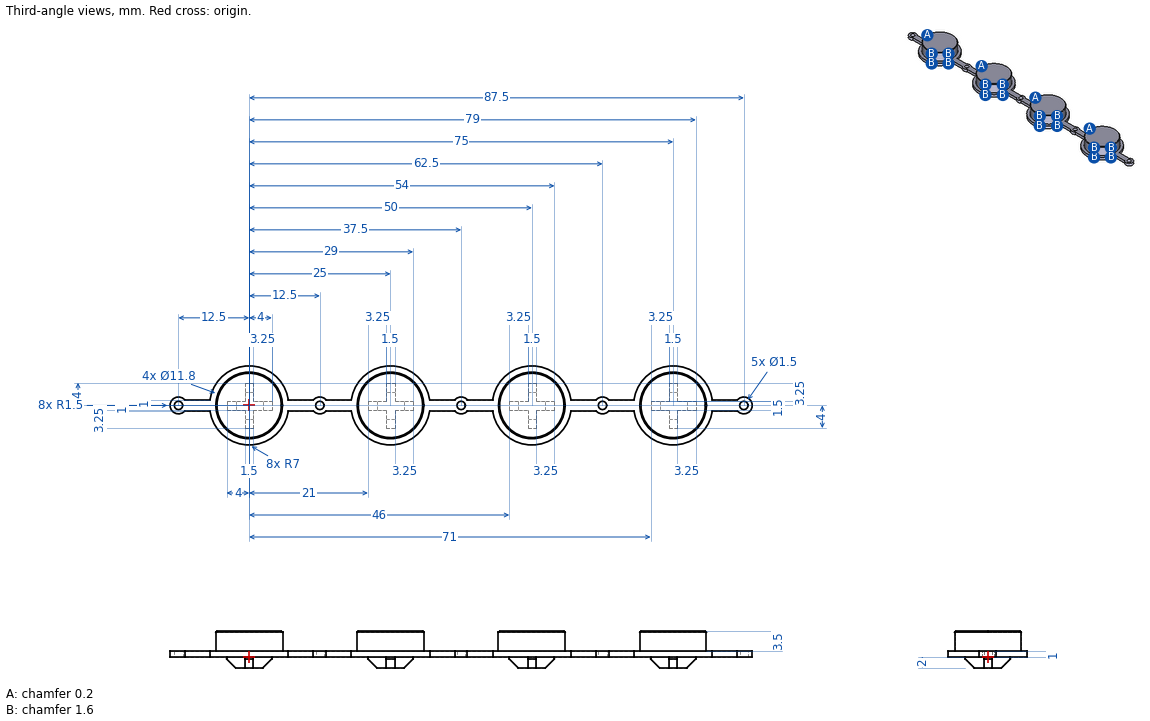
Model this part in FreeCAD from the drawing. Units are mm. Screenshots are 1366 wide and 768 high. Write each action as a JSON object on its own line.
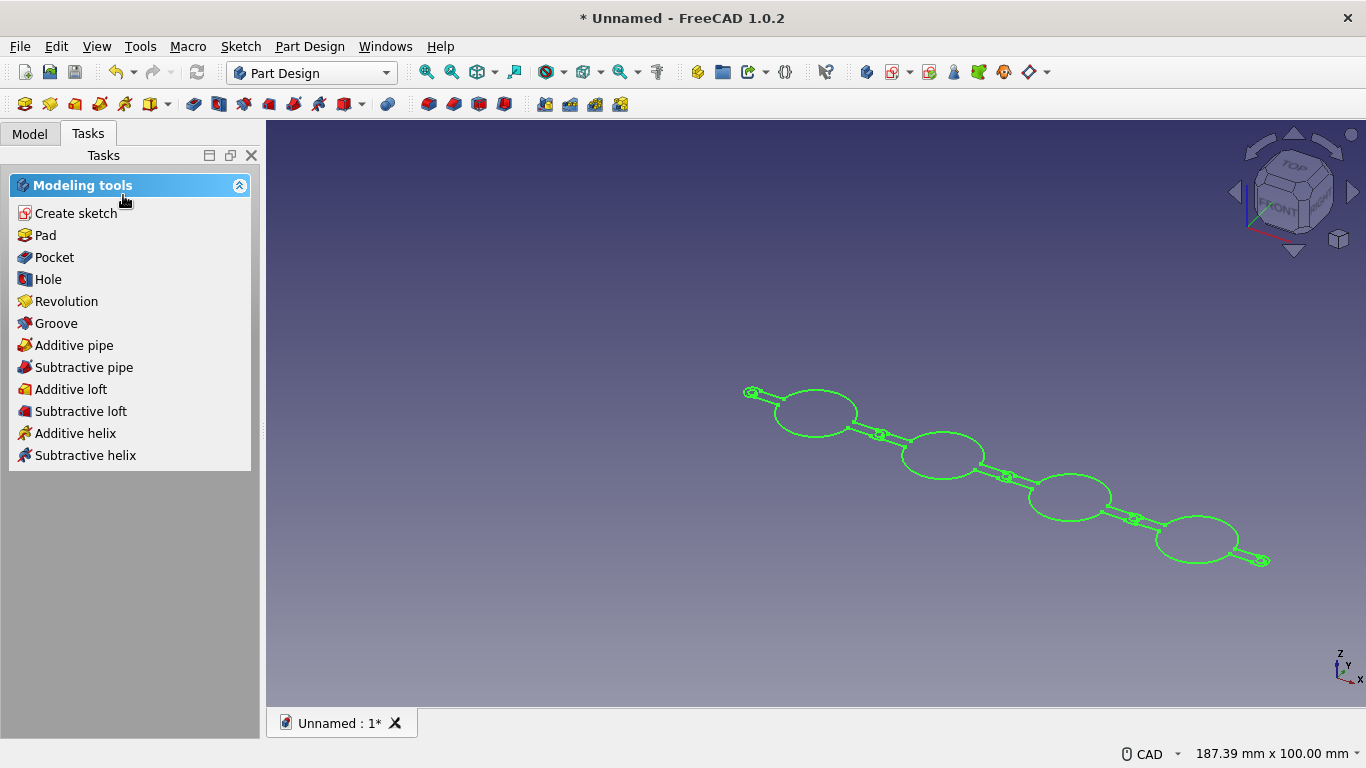
{"action": "left_click", "coordinate": [25, 104]}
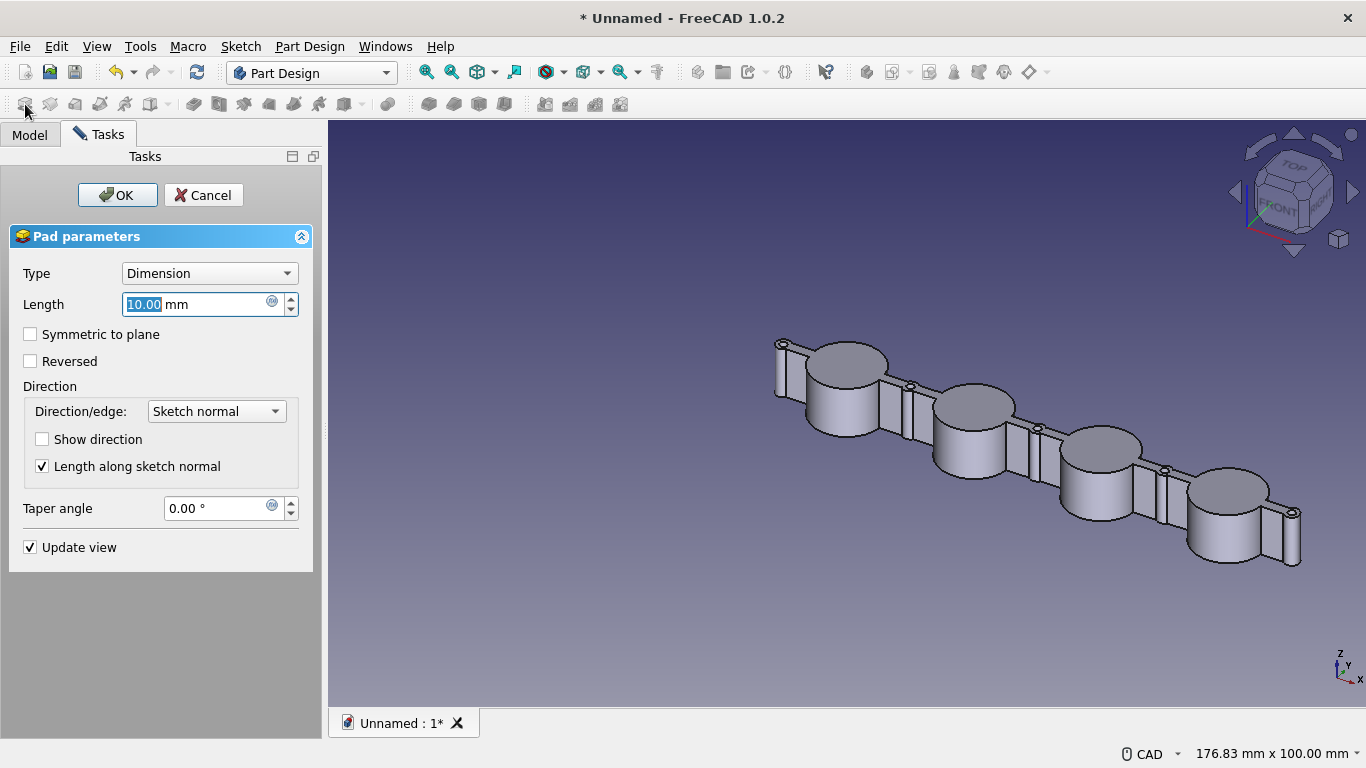
{"action": "type", "text": "1"}
{"action": "key", "text": "Tab"}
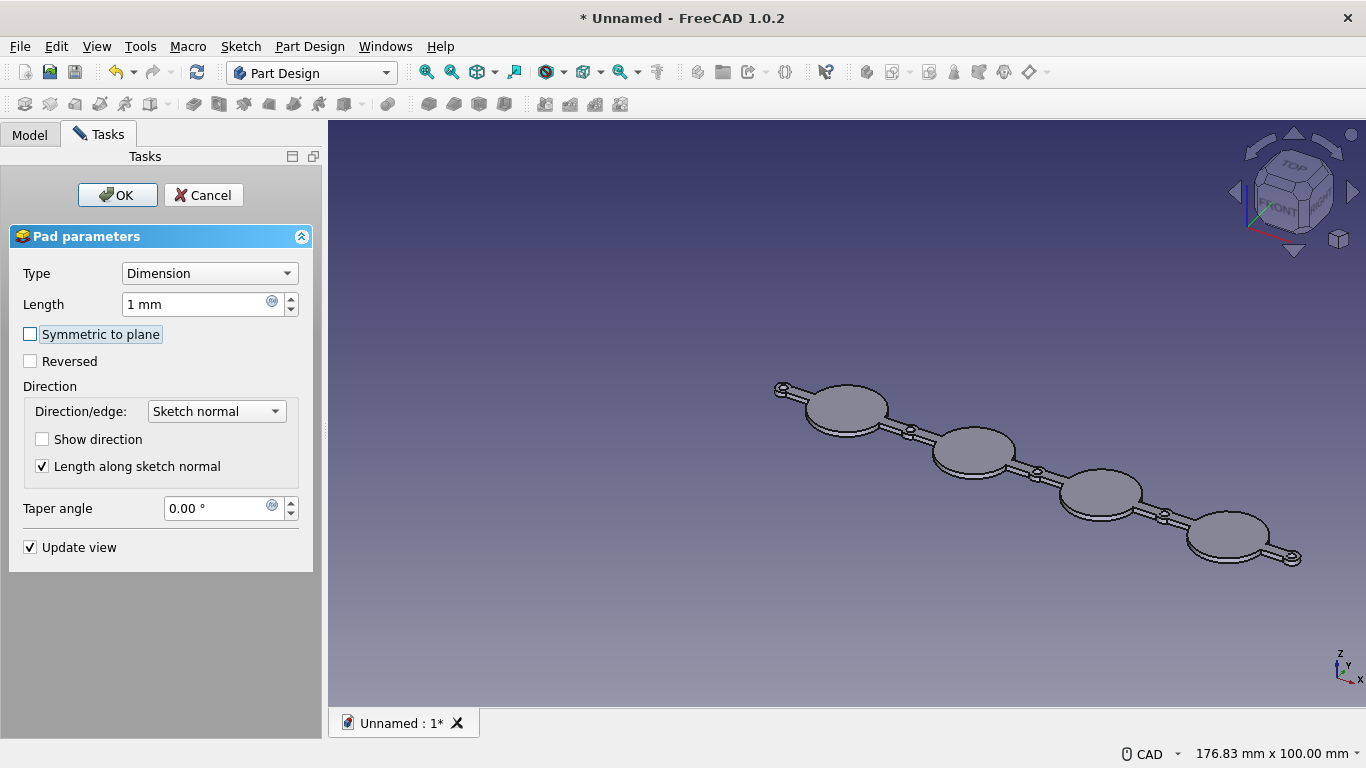
{"action": "left_click", "coordinate": [118, 195]}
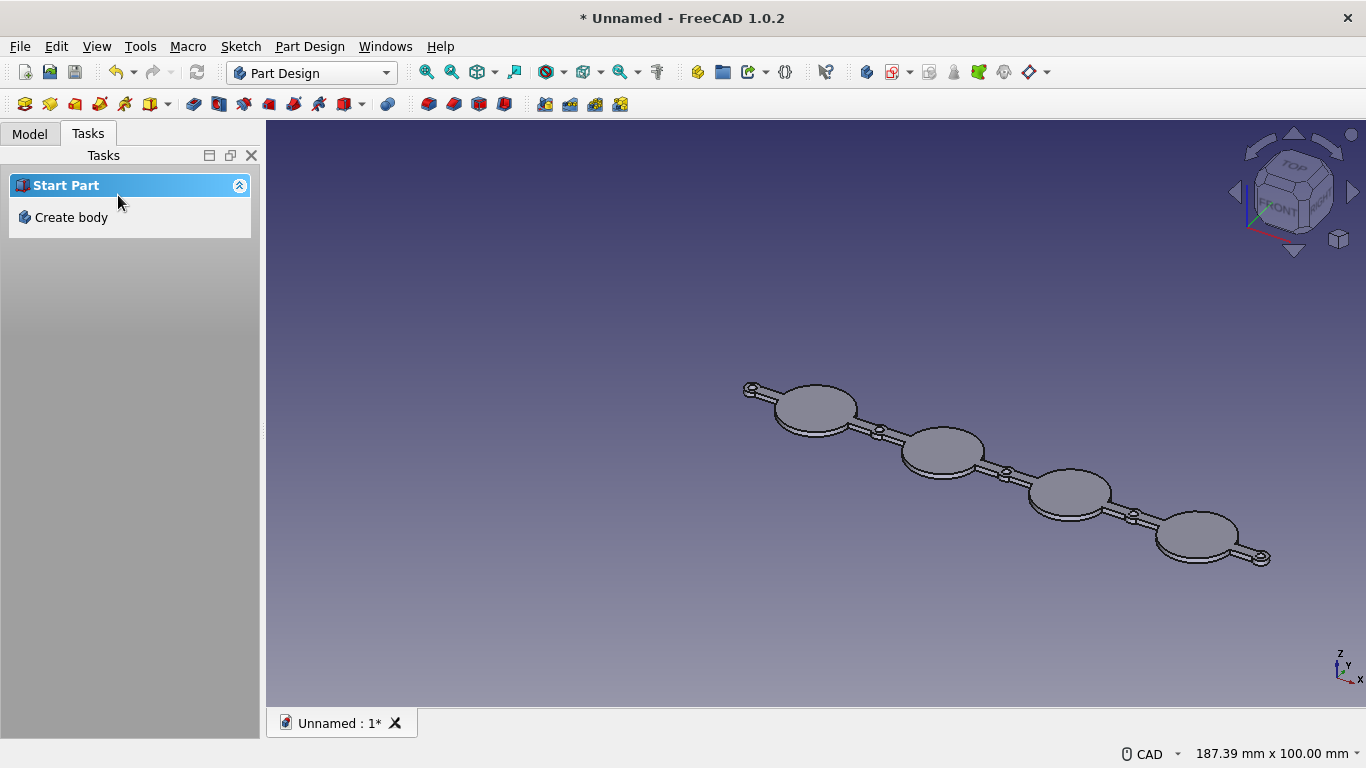
{"action": "left_click", "coordinate": [1081, 496]}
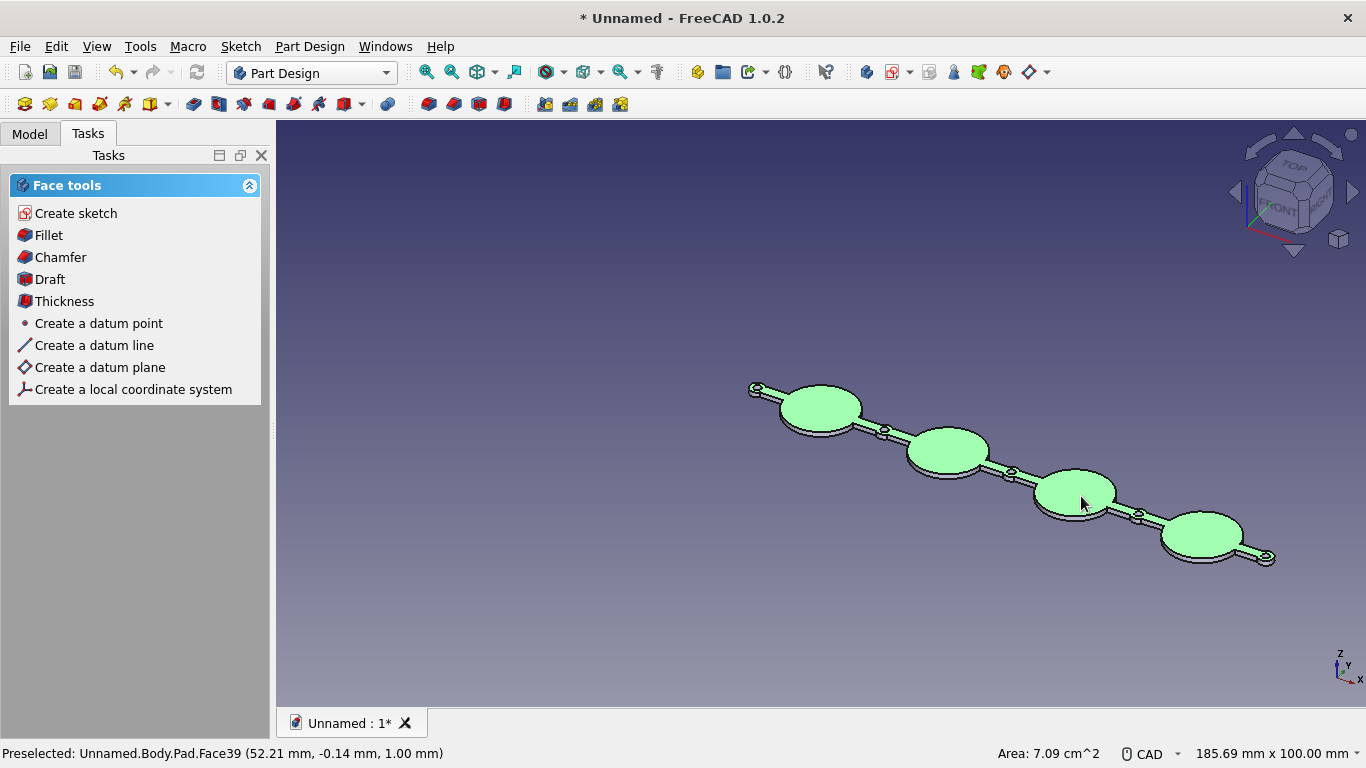
{"action": "left_click", "coordinate": [892, 72]}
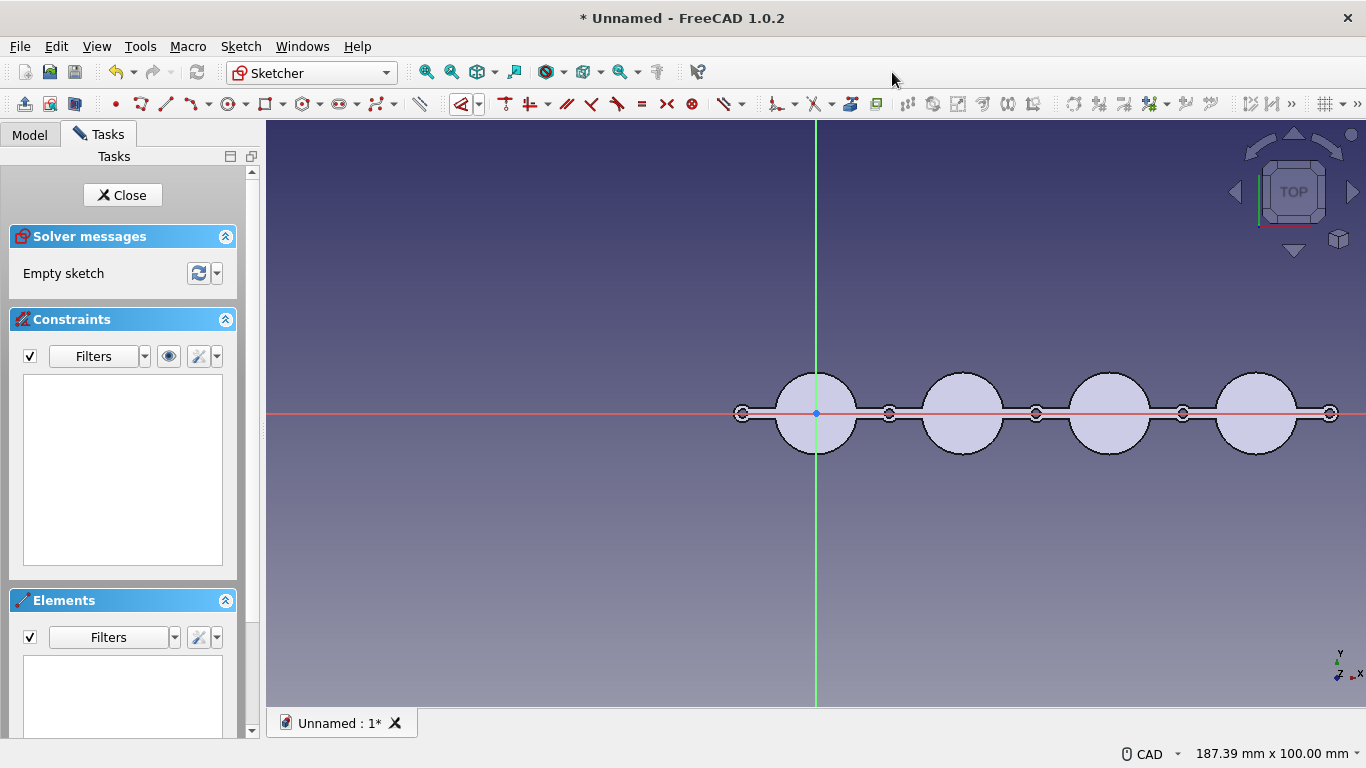
{"action": "scroll", "coordinate": [294, 413], "scroll_direction": "down", "scroll_amount": 1}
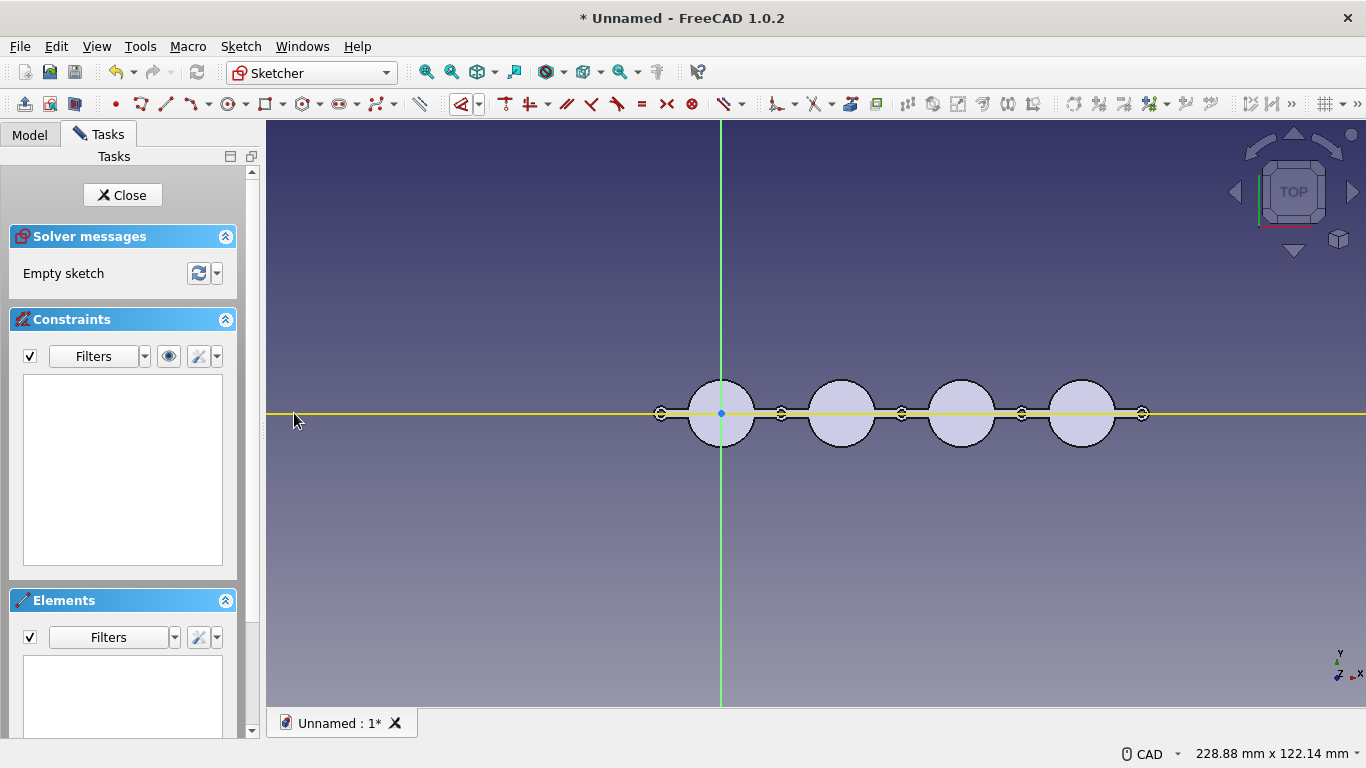
{"action": "scroll", "coordinate": [1201, 413], "scroll_direction": "up", "scroll_amount": 2}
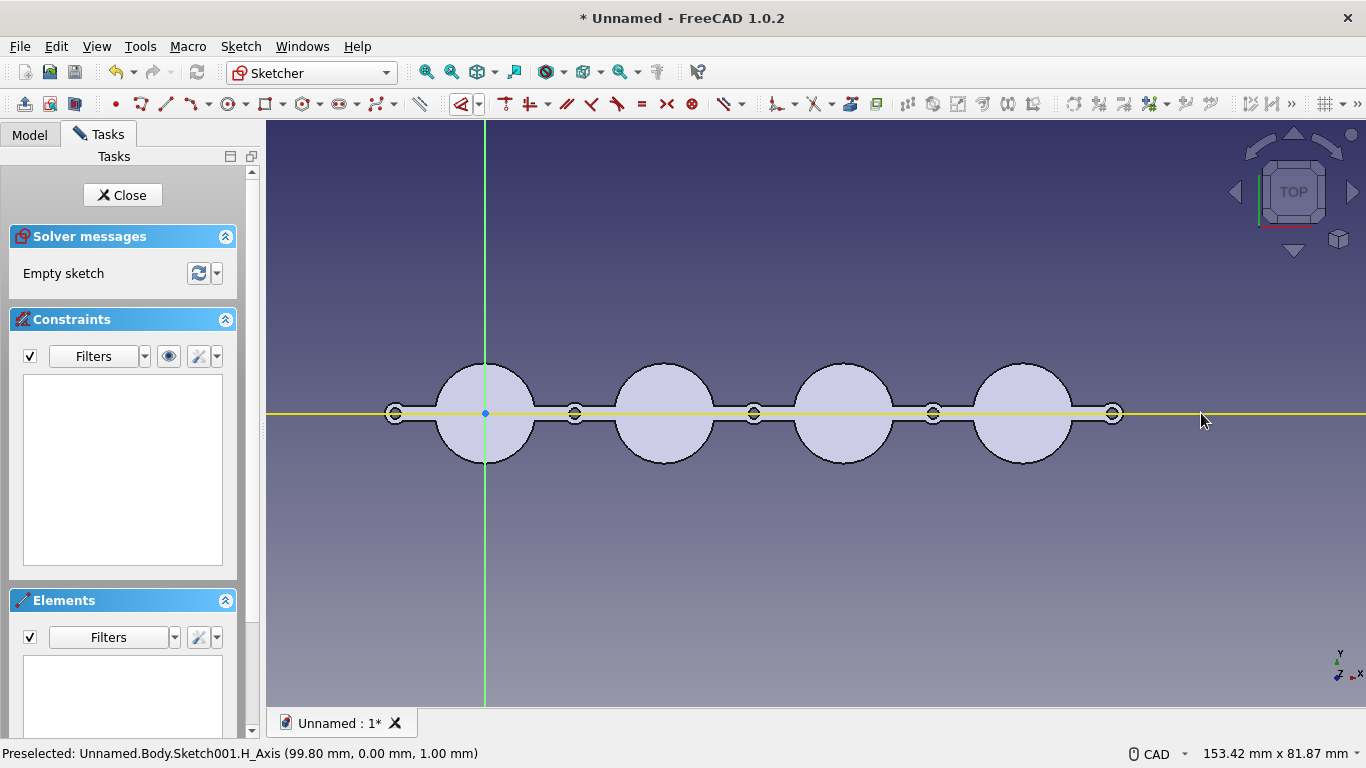
{"action": "key", "text": "g c"}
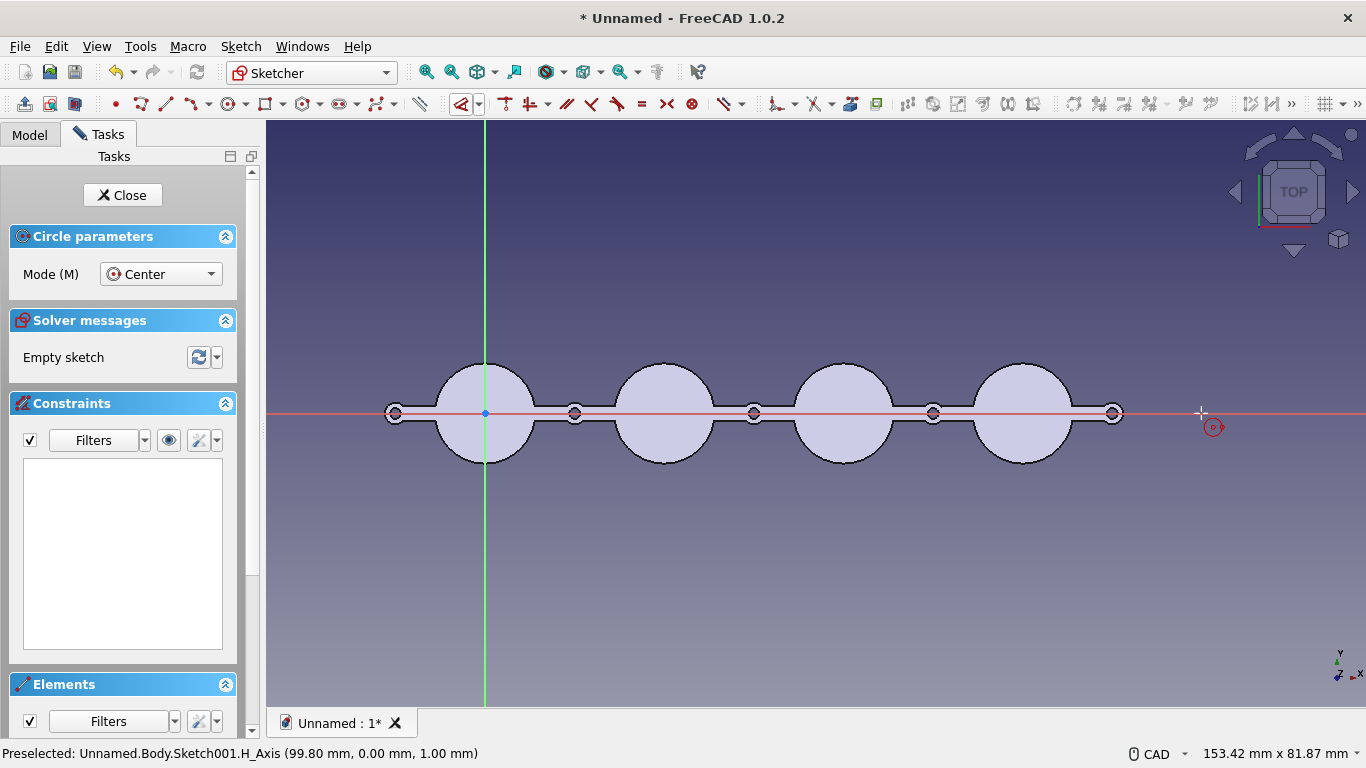
{"action": "left_click", "coordinate": [485, 414]}
{"action": "left_click", "coordinate": [515, 384]}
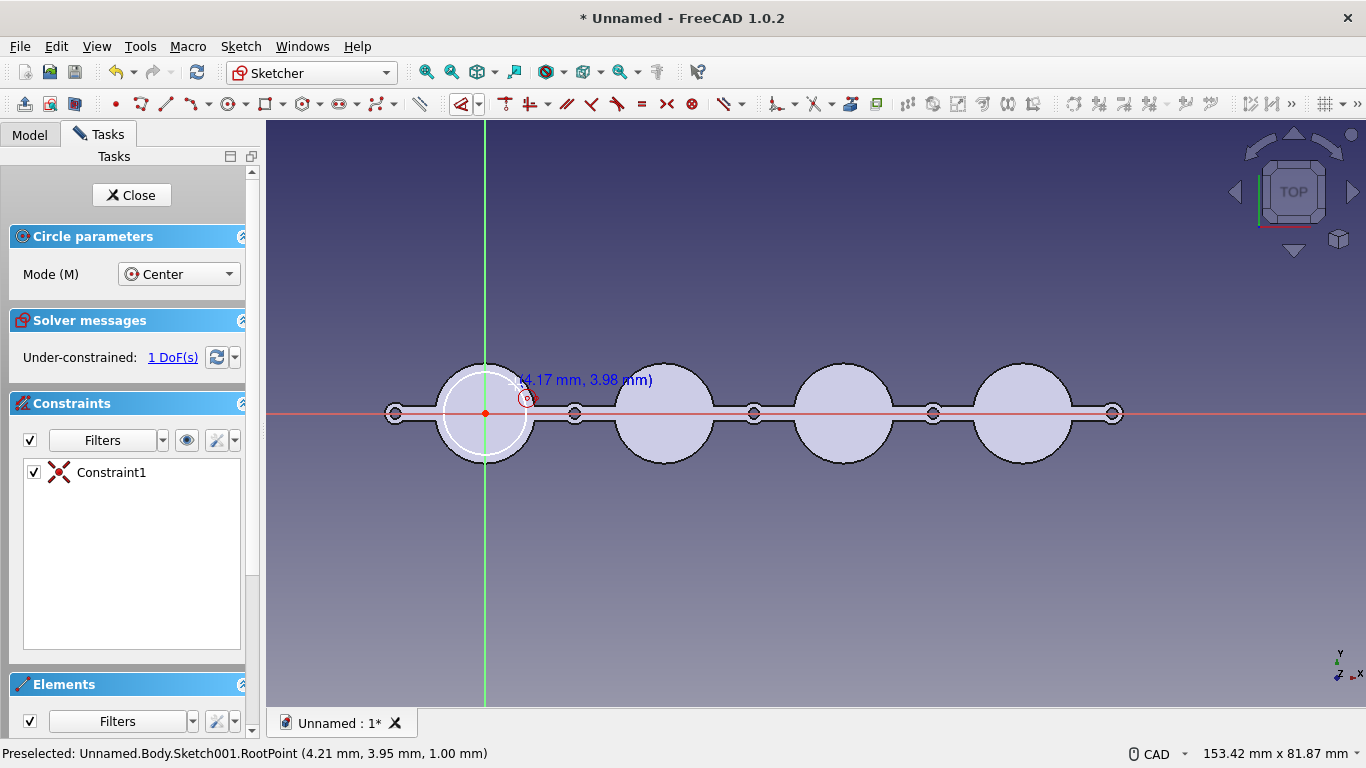
{"action": "left_click", "coordinate": [664, 414]}
{"action": "left_click", "coordinate": [694, 384]}